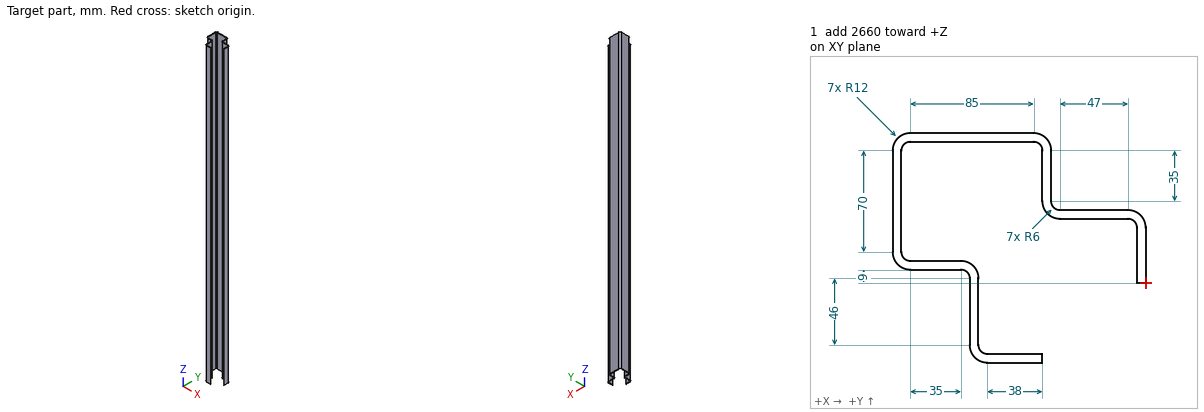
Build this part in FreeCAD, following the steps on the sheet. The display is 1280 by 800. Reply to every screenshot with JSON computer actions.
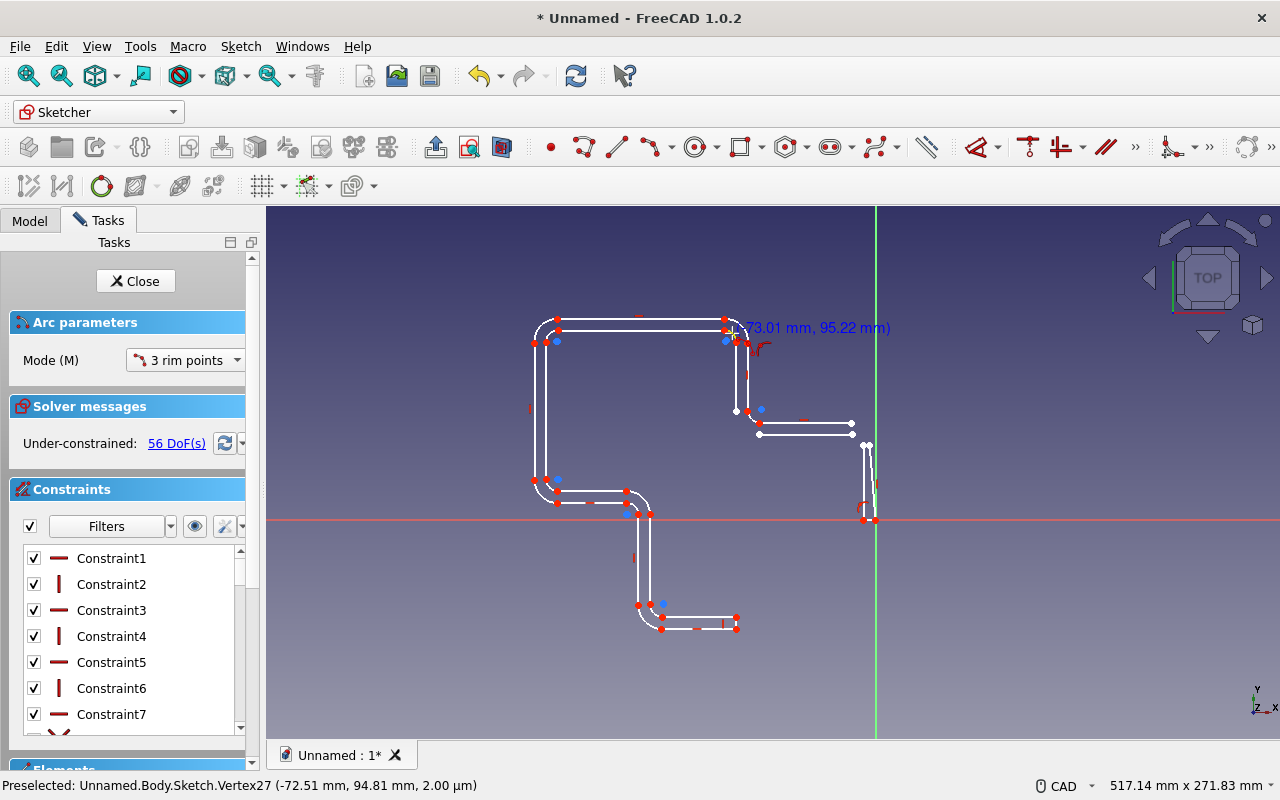
{"action": "scroll", "coordinate": [736, 410], "scroll_direction": "up", "scroll_amount": 2}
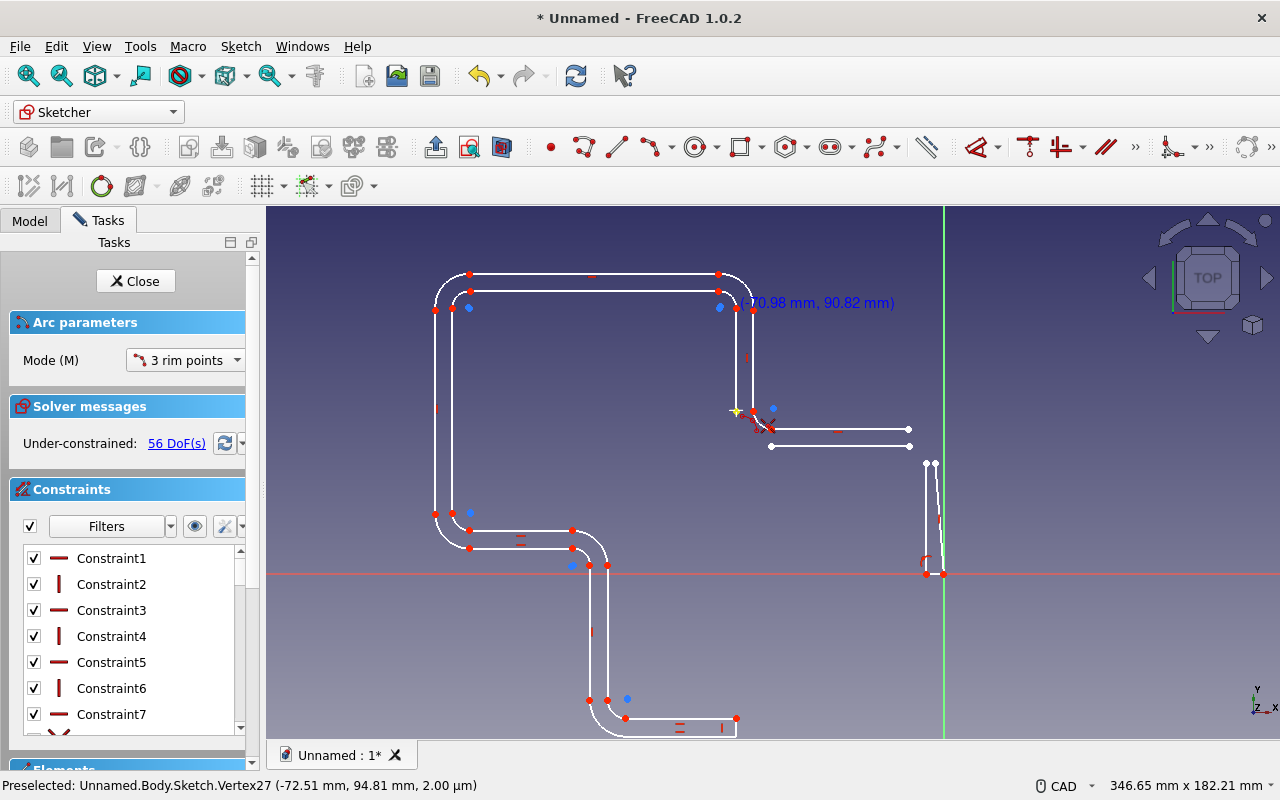
{"action": "left_click", "coordinate": [736, 411]}
{"action": "left_click", "coordinate": [771, 446]}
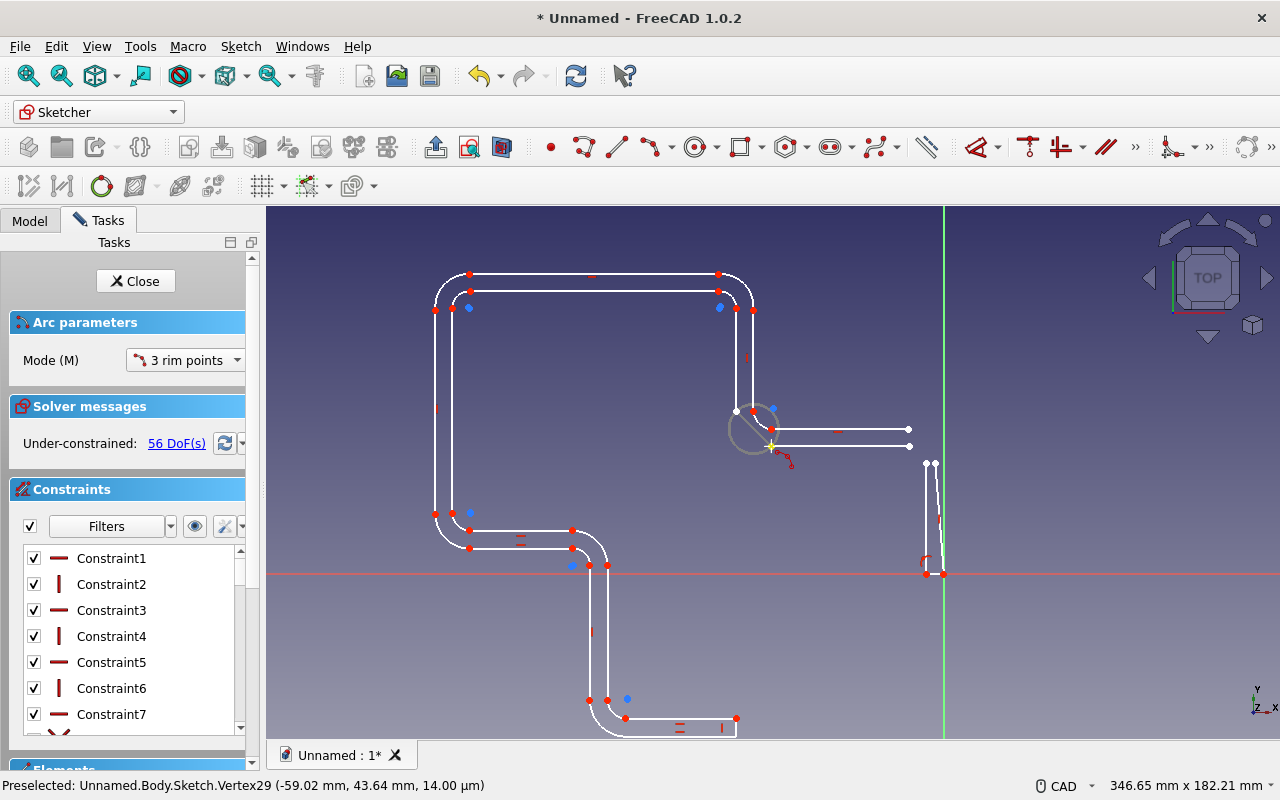
{"action": "scroll", "coordinate": [747, 435], "scroll_direction": "up", "scroll_amount": 3}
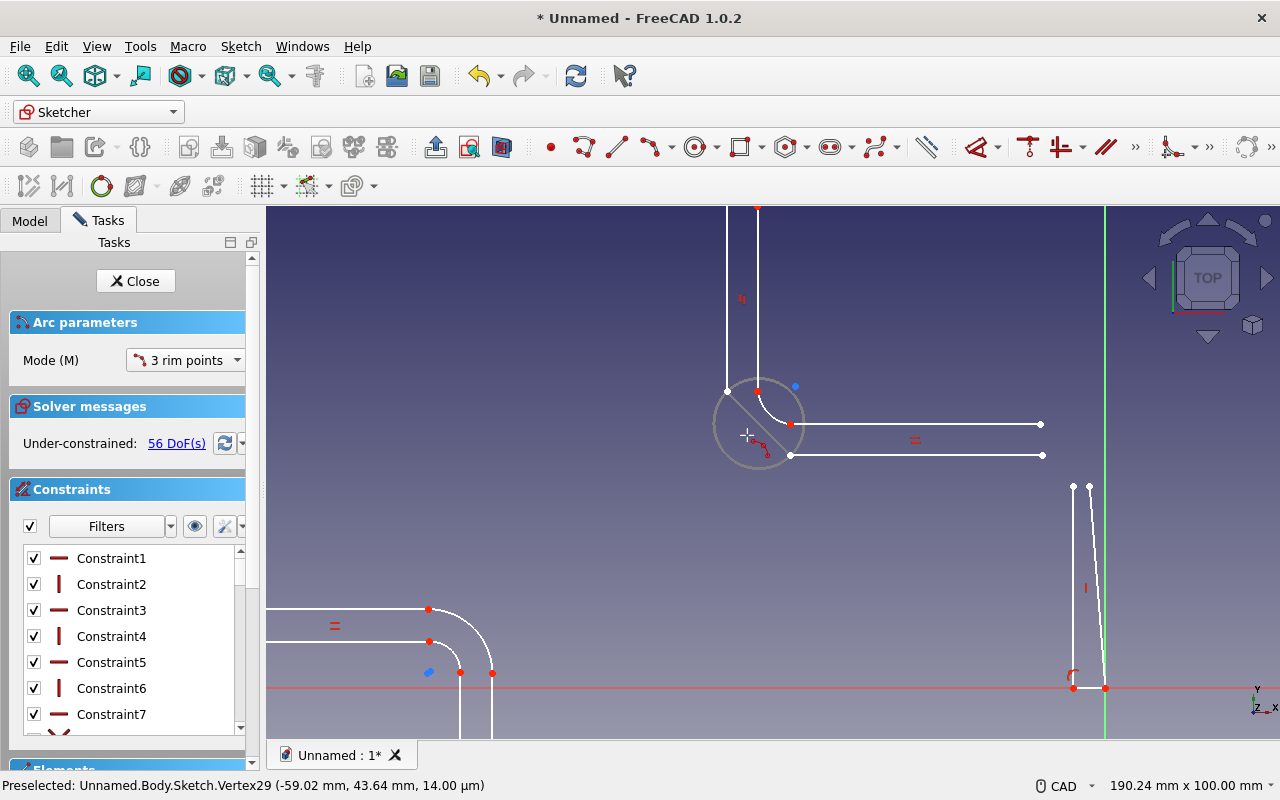
{"action": "left_click", "coordinate": [746, 435]}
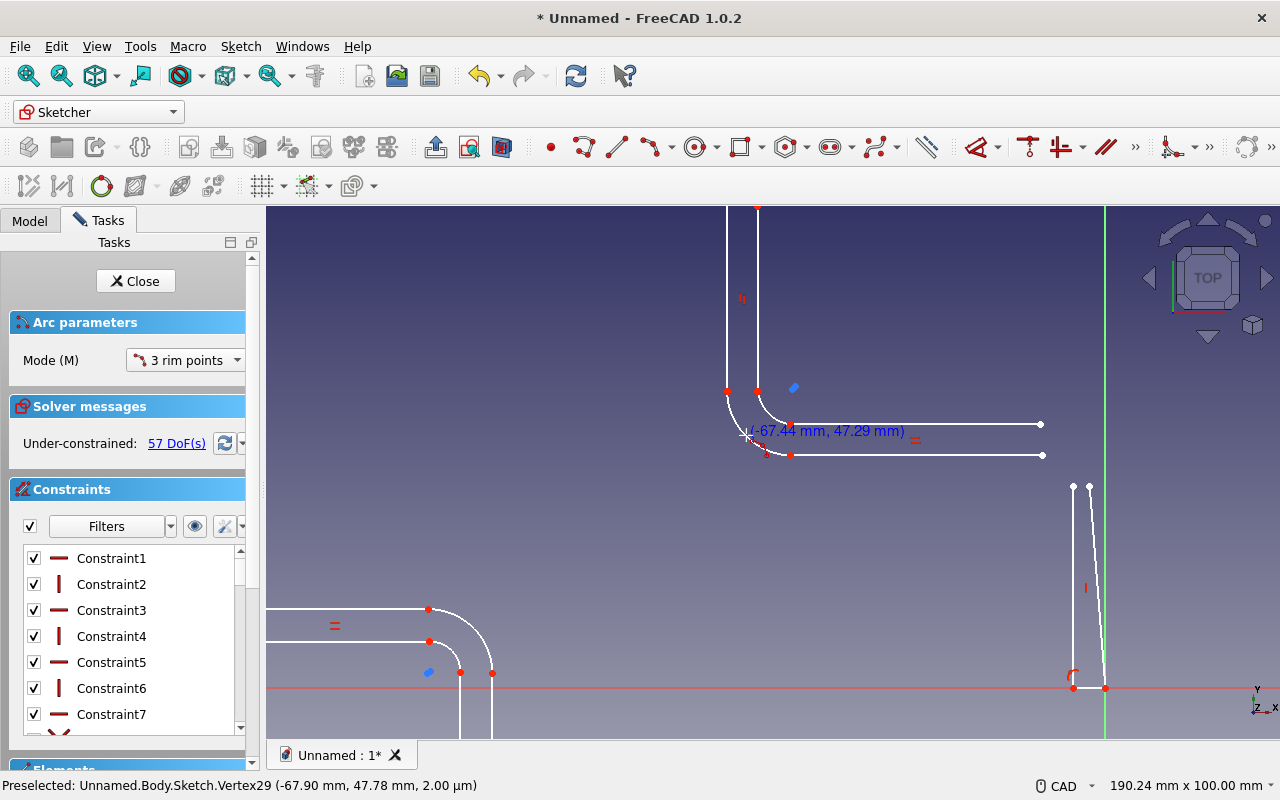
{"action": "left_click", "coordinate": [1042, 455]}
{"action": "left_click", "coordinate": [1073, 486]}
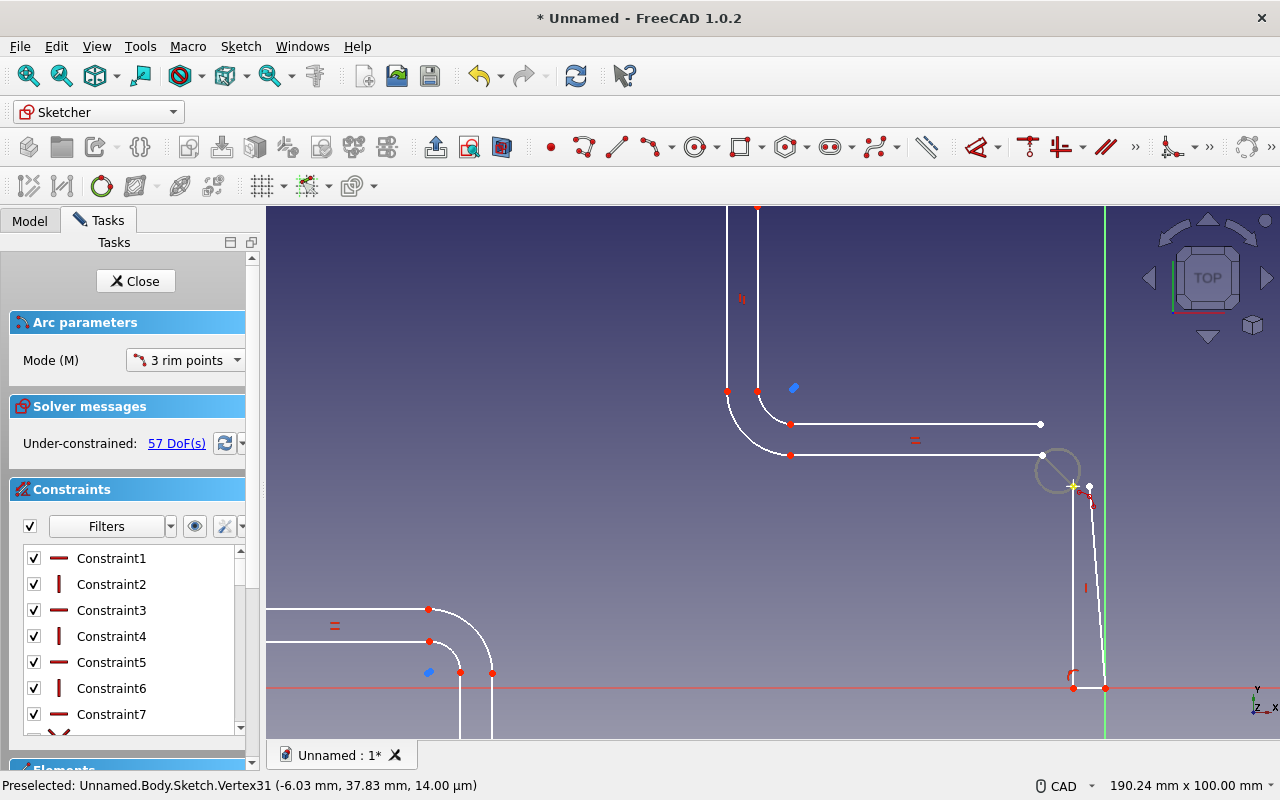
{"action": "scroll", "coordinate": [1064, 463], "scroll_direction": "up", "scroll_amount": 3}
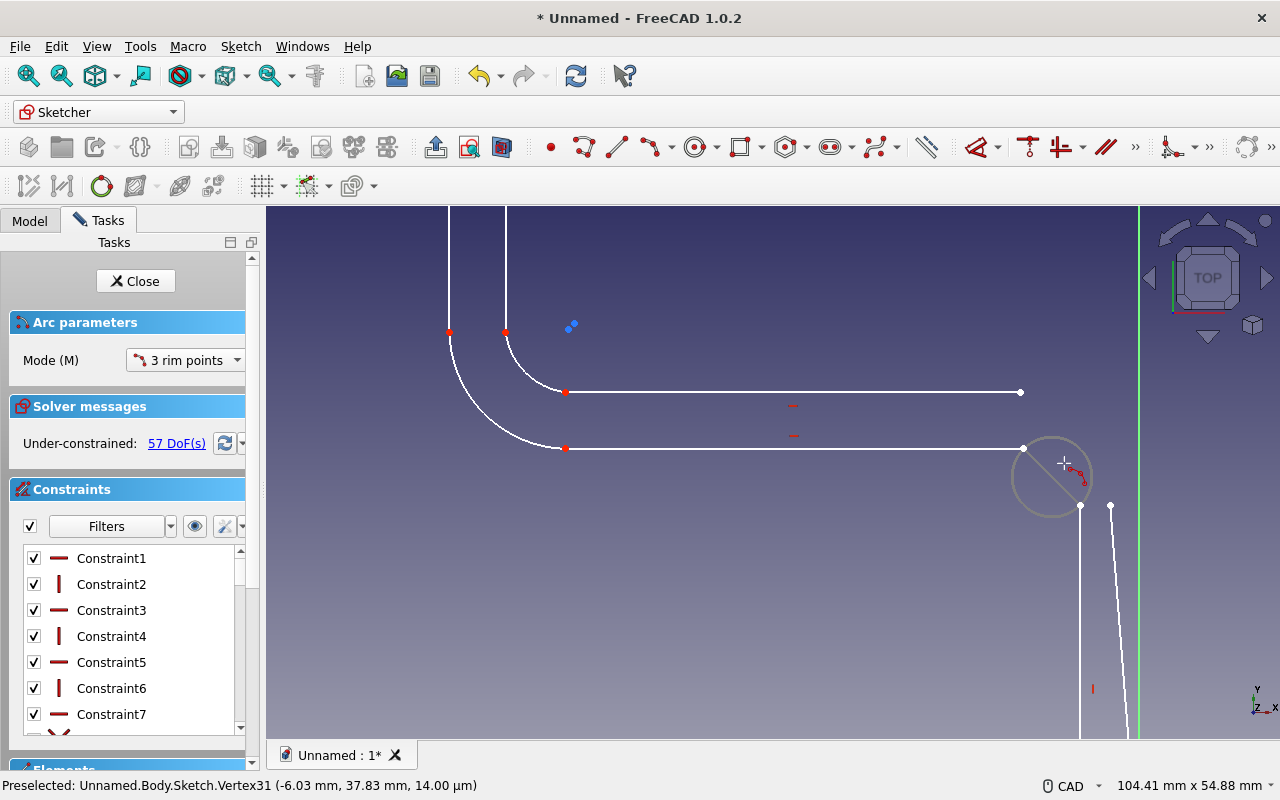
{"action": "left_click", "coordinate": [1064, 462]}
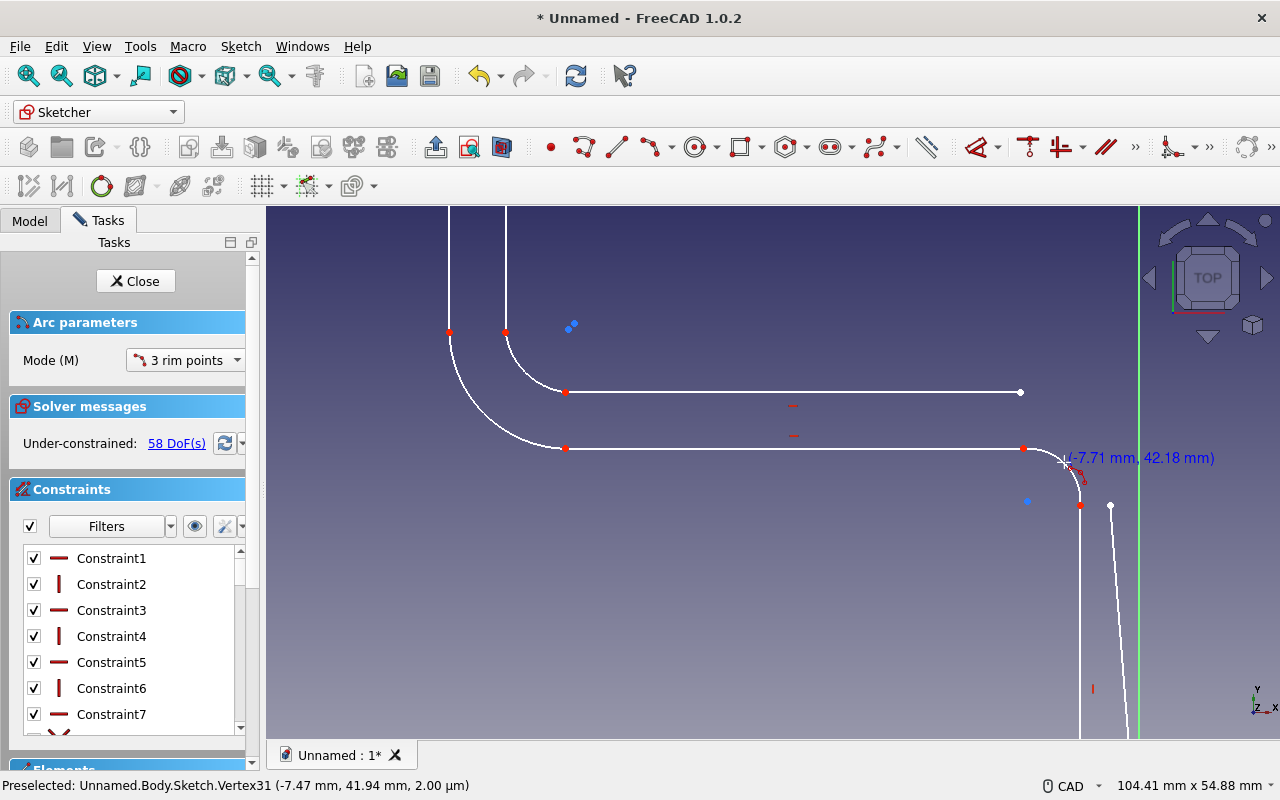
{"action": "scroll", "coordinate": [808, 430], "scroll_direction": "down", "scroll_amount": 8}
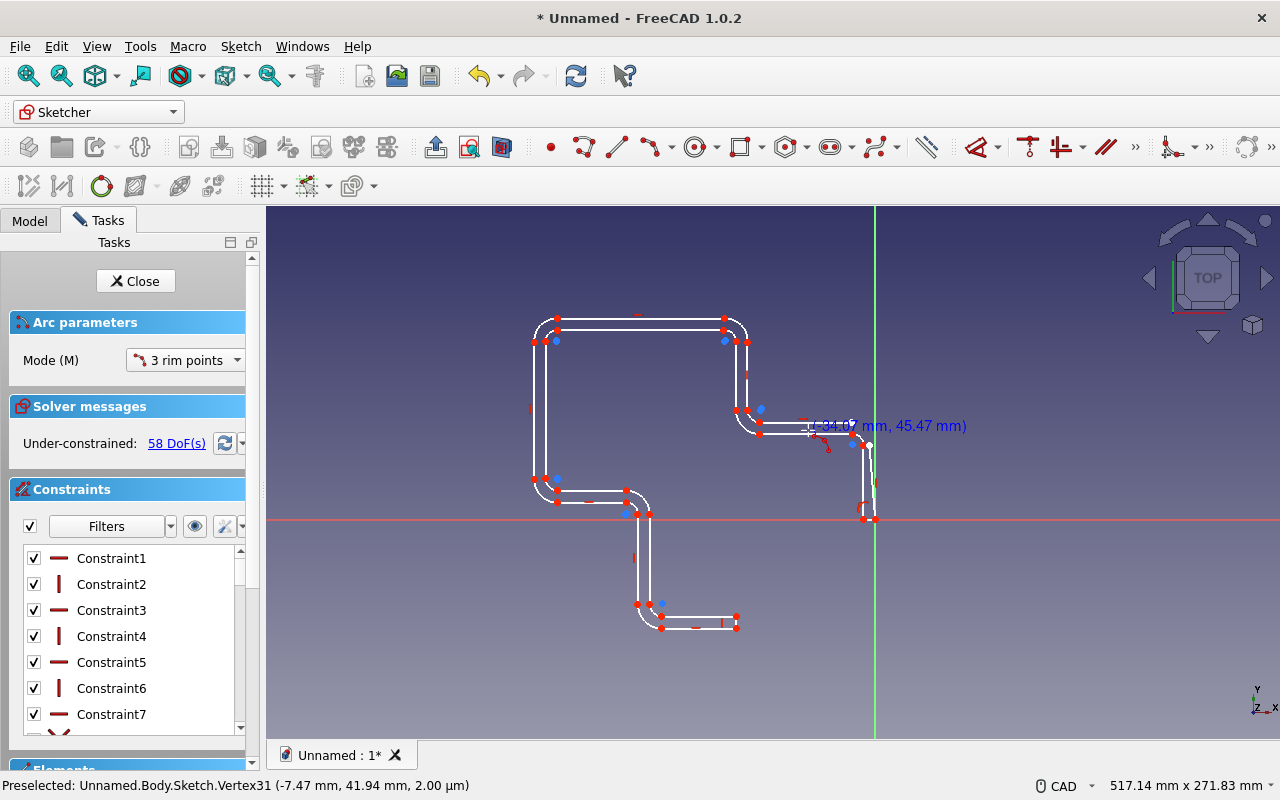
{"action": "scroll", "coordinate": [875, 445], "scroll_direction": "up", "scroll_amount": 2}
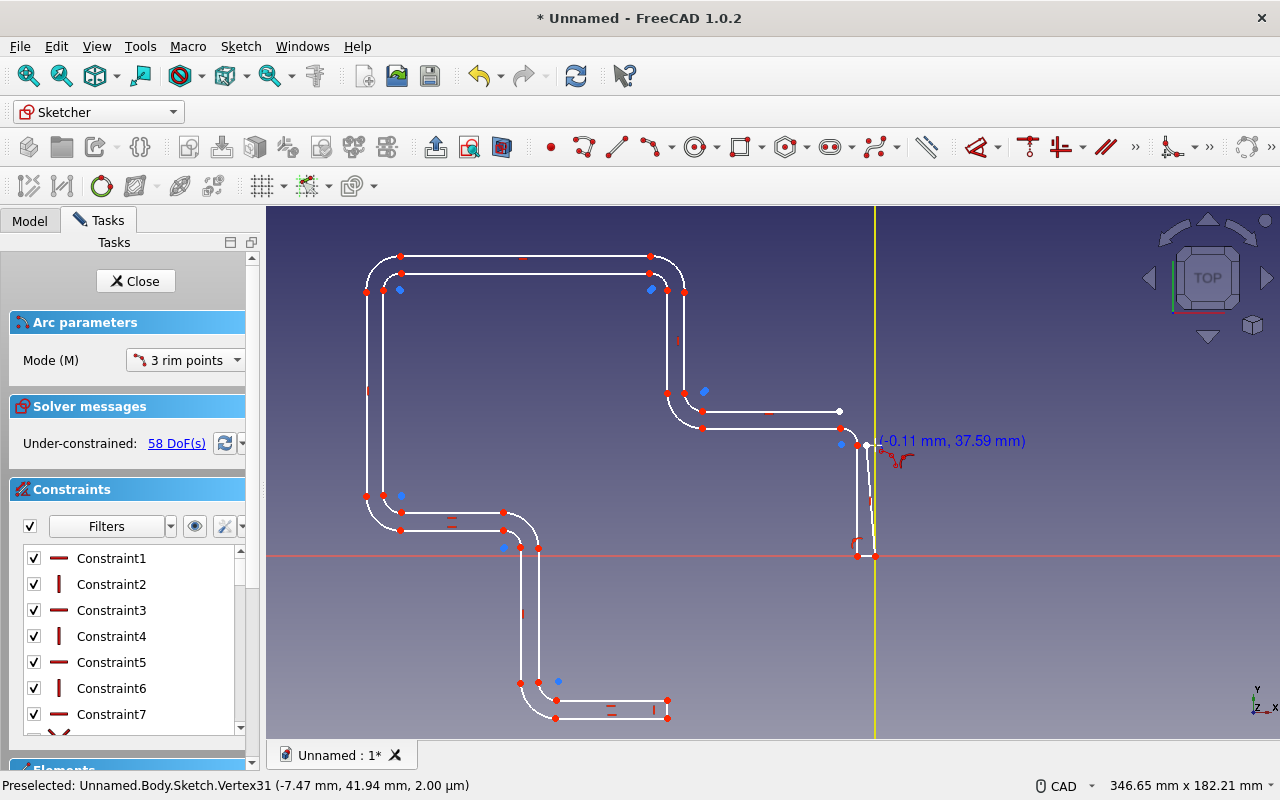
{"action": "left_click", "coordinate": [866, 446]}
{"action": "left_click", "coordinate": [840, 412]}